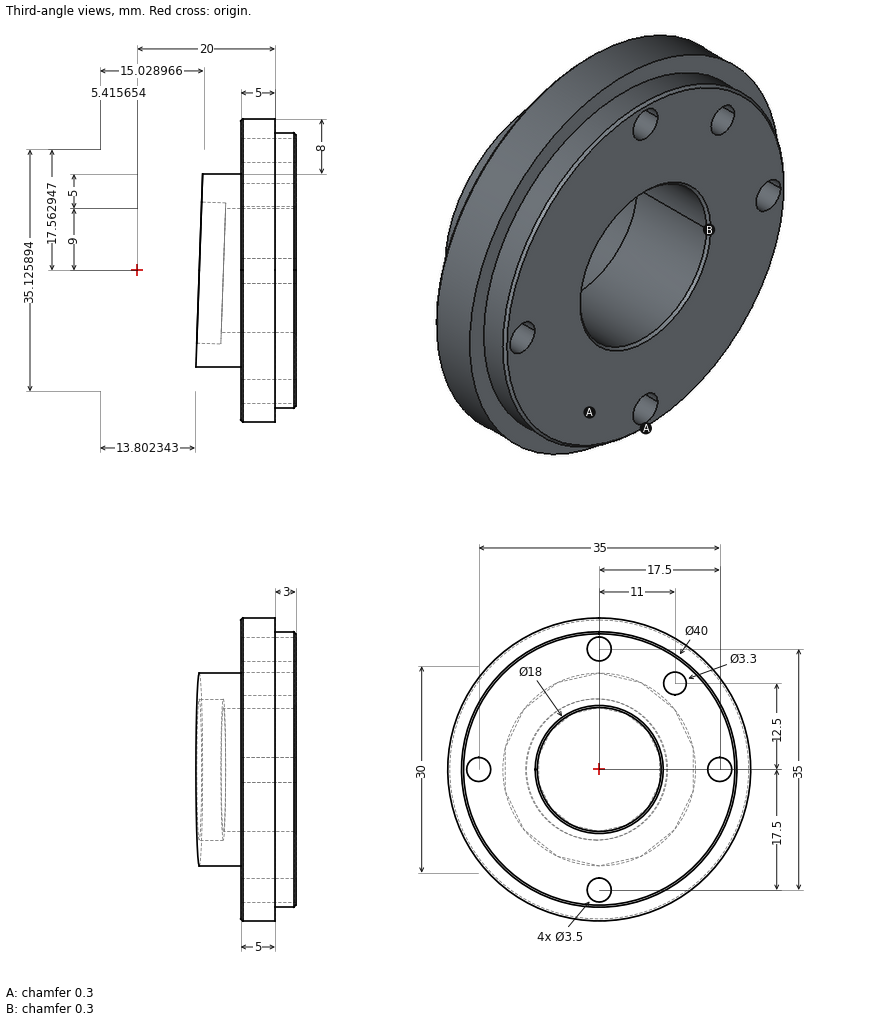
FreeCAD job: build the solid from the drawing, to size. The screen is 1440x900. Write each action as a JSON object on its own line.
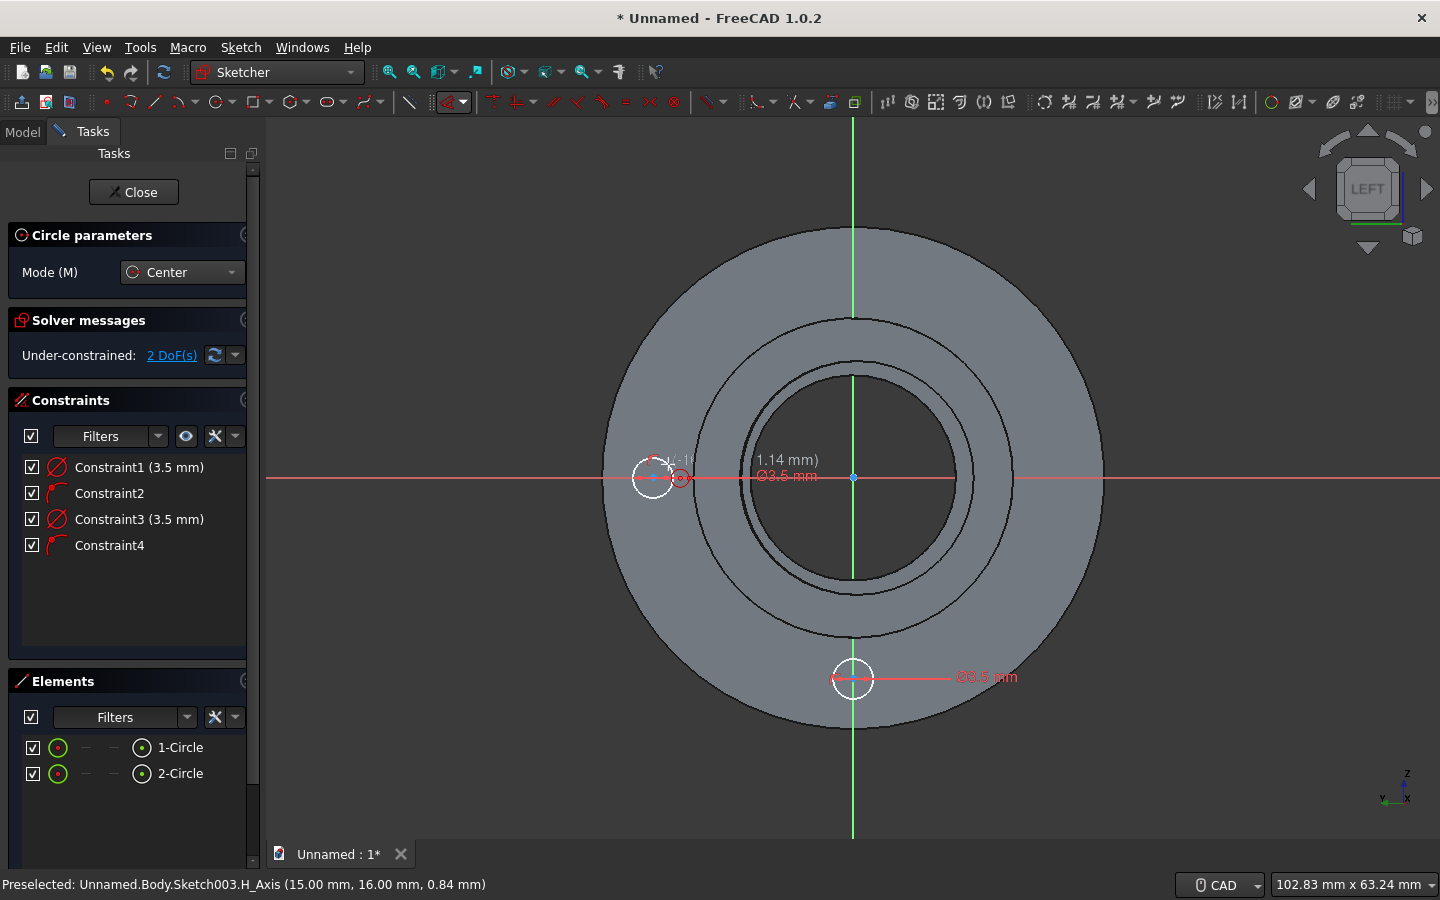
{"action": "left_click", "coordinate": [853, 278]}
{"action": "mouse_move", "coordinate": [867, 264]}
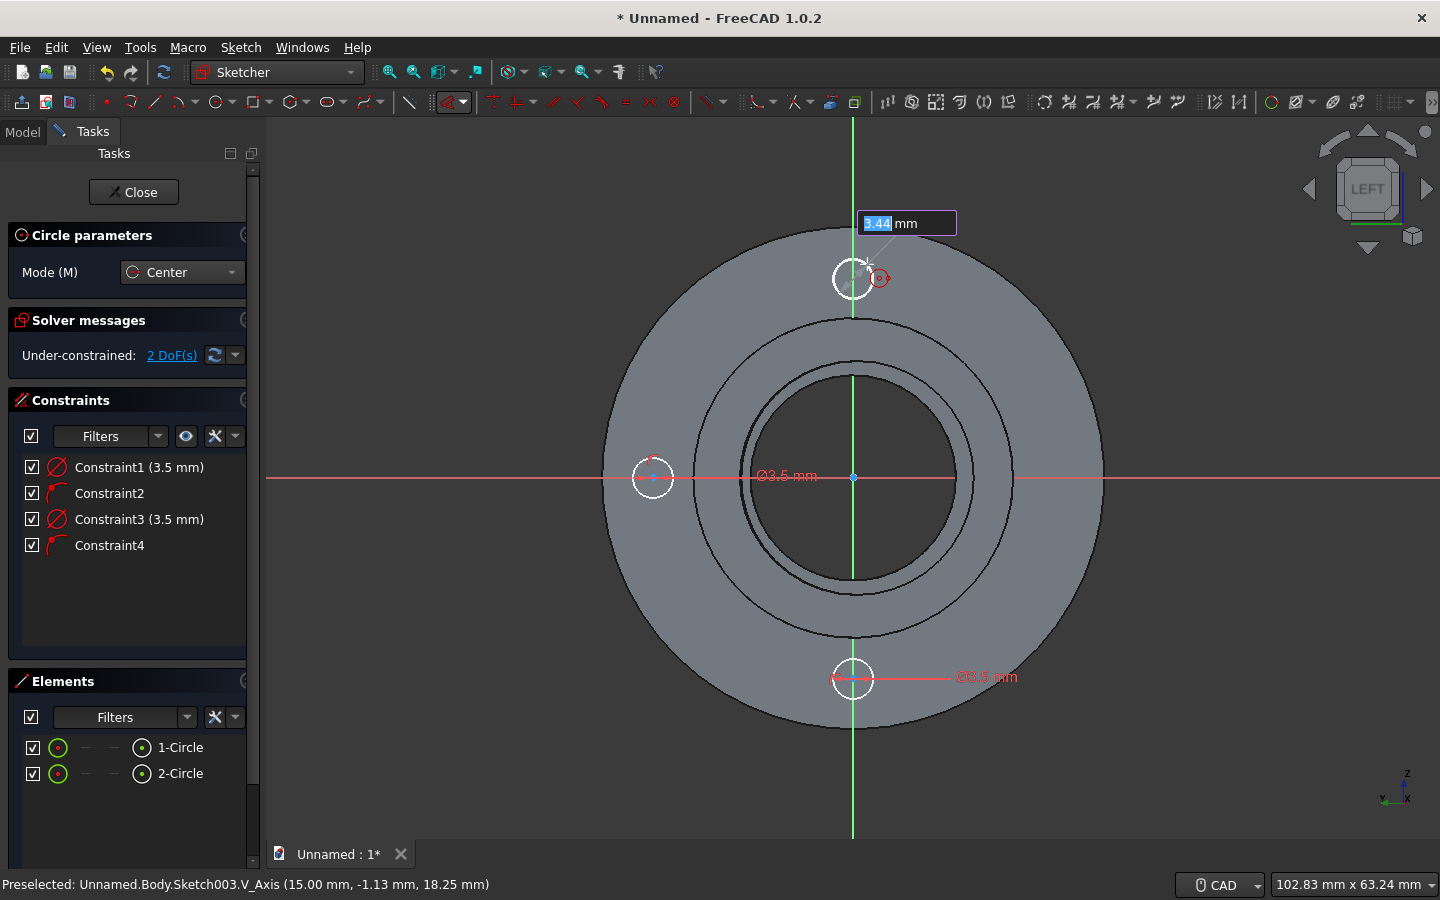
{"action": "type", "text": "3.5"}
{"action": "key", "text": "Return"}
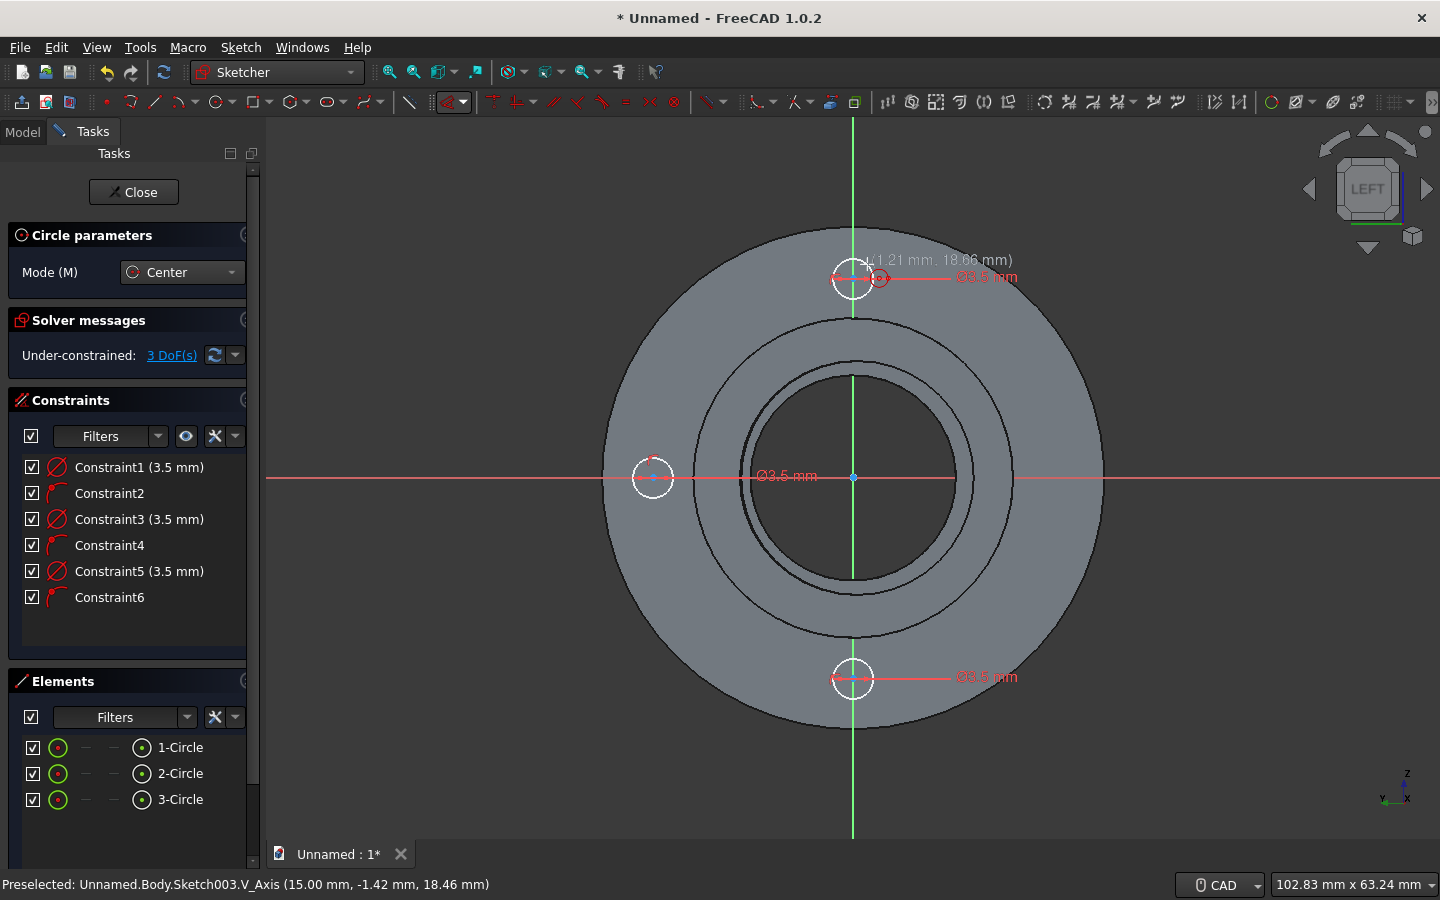
{"action": "left_click", "coordinate": [1053, 478]}
{"action": "mouse_move", "coordinate": [1067, 464]}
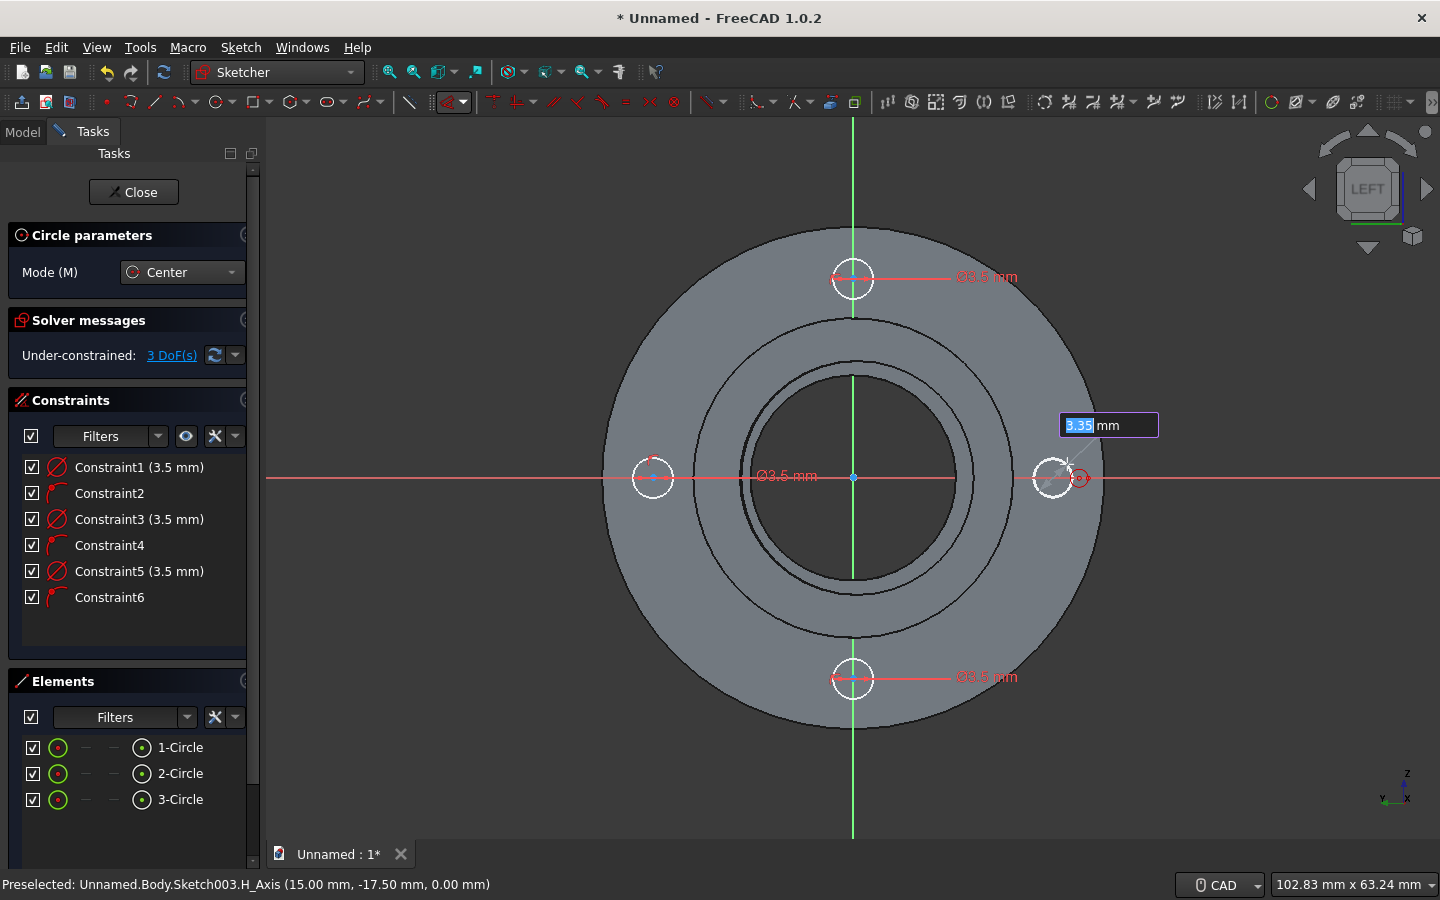
{"action": "type", "text": "3.5"}
{"action": "key", "text": "Return"}
{"action": "key", "text": "Escape"}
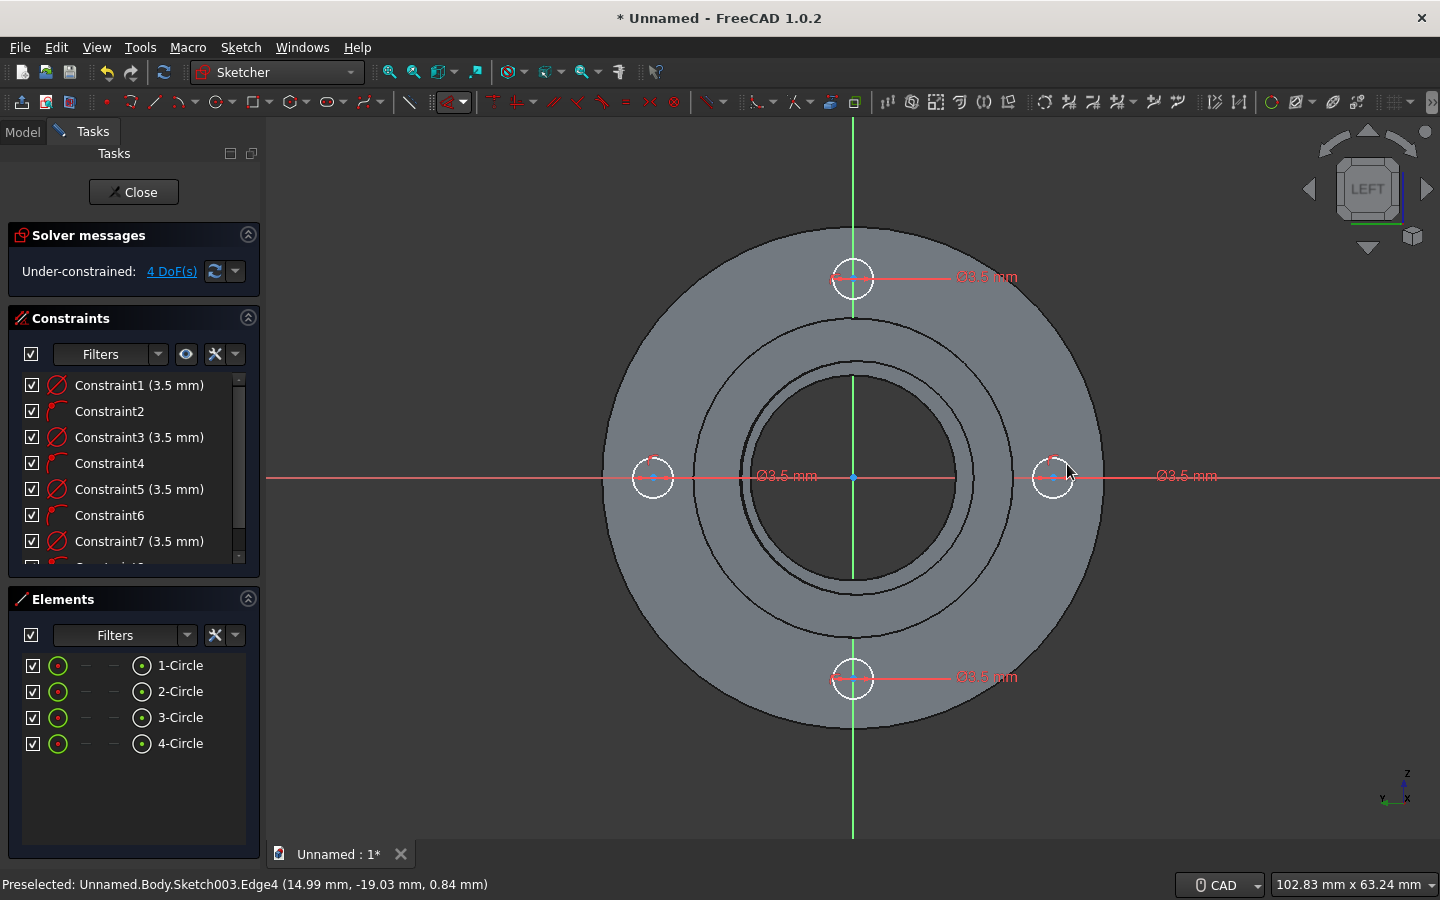
{"action": "left_click", "coordinate": [853, 679]}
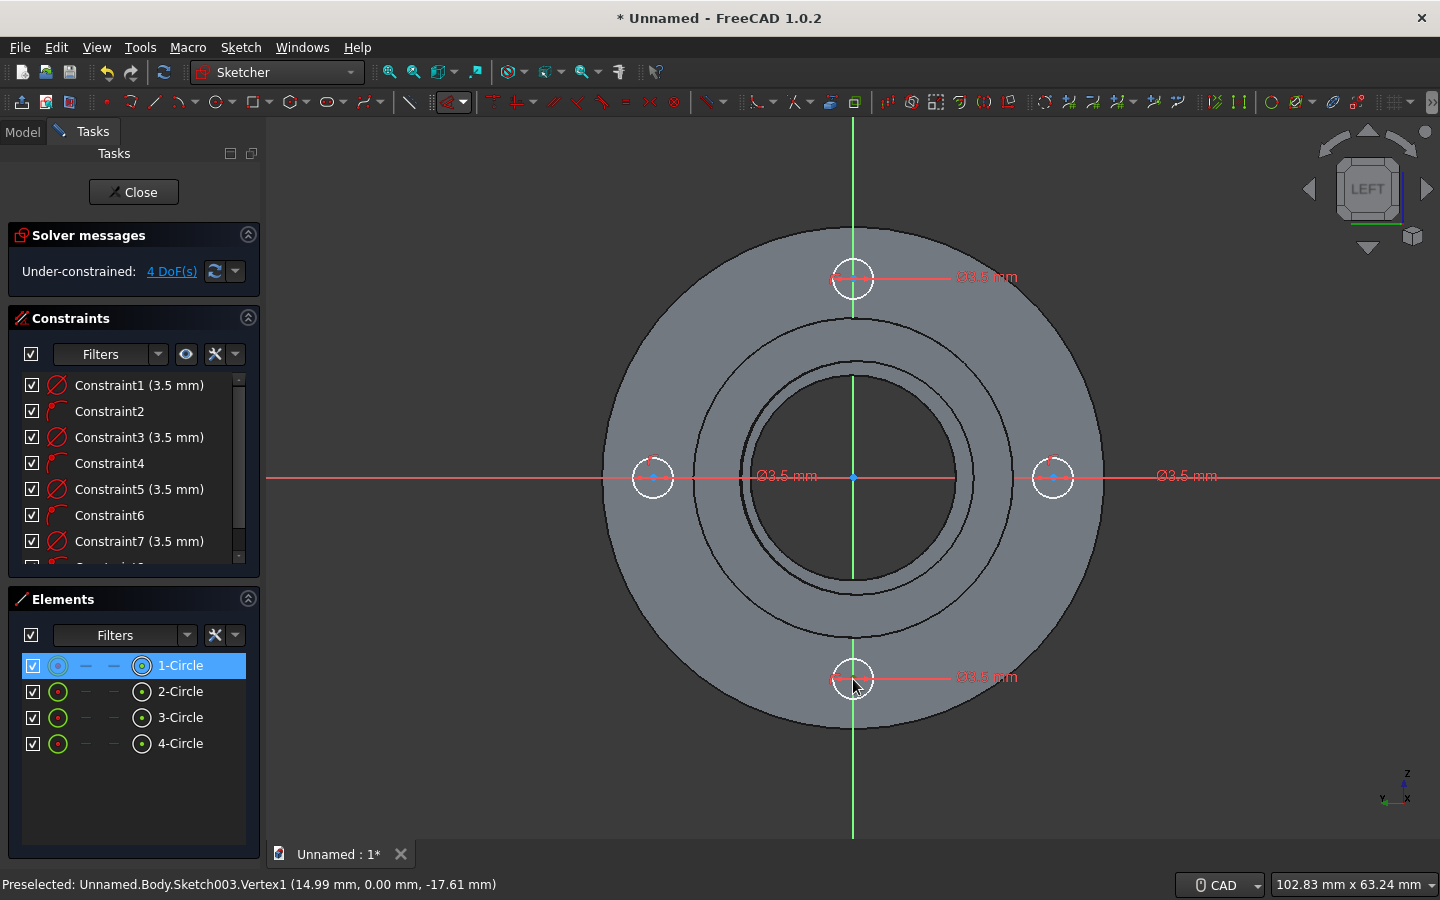
{"action": "left_click", "coordinate": [853, 279]}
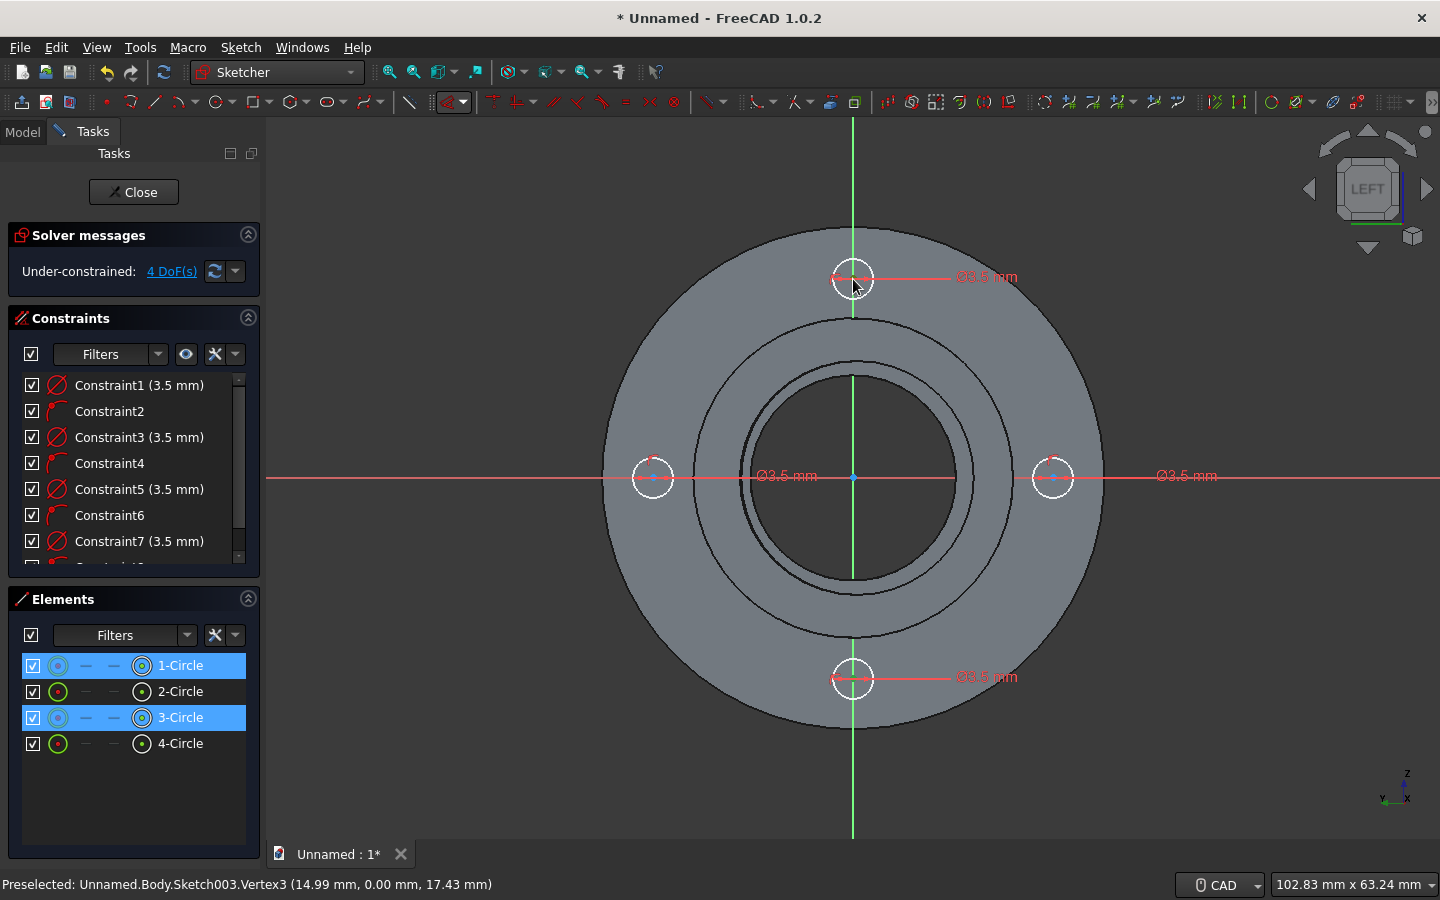
{"action": "key", "text": "i"}